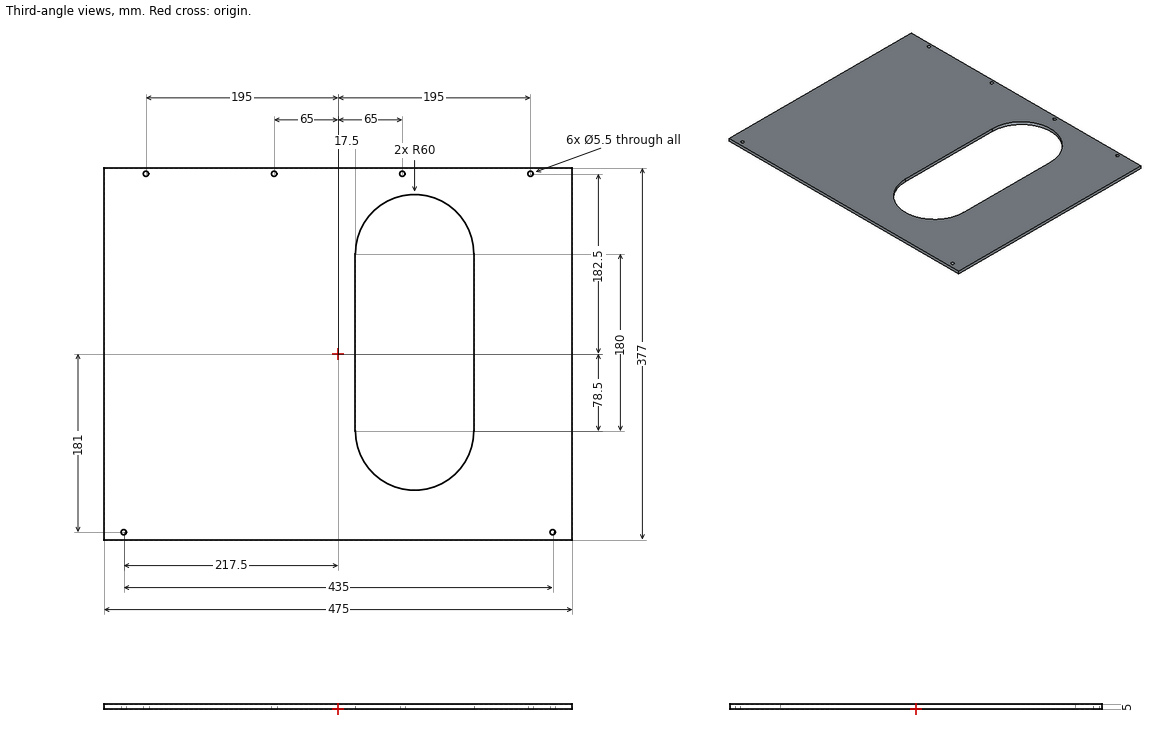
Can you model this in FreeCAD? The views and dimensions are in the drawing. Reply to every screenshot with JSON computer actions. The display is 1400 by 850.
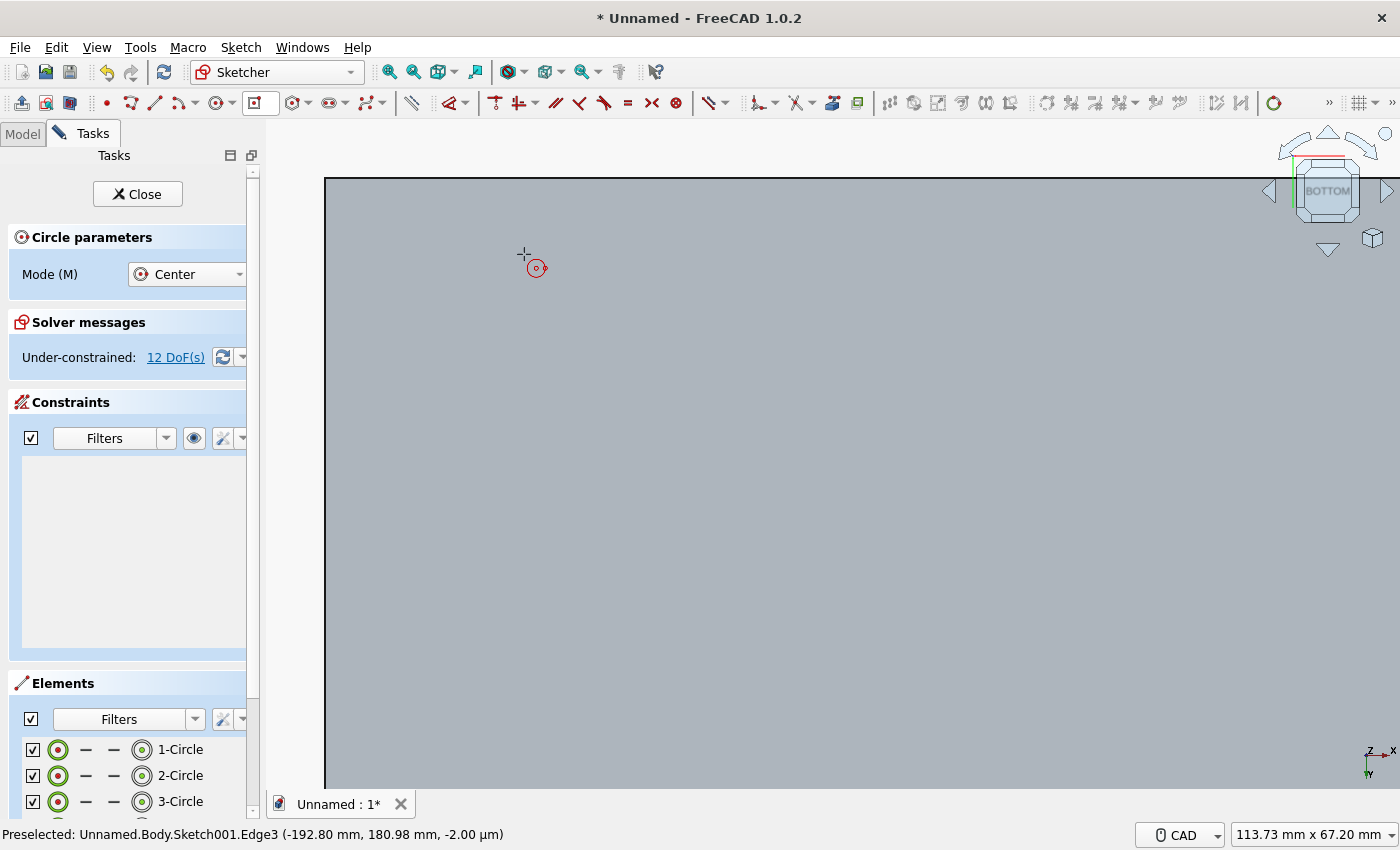
{"action": "scroll", "coordinate": [524, 253], "scroll_direction": "down", "scroll_amount": 11}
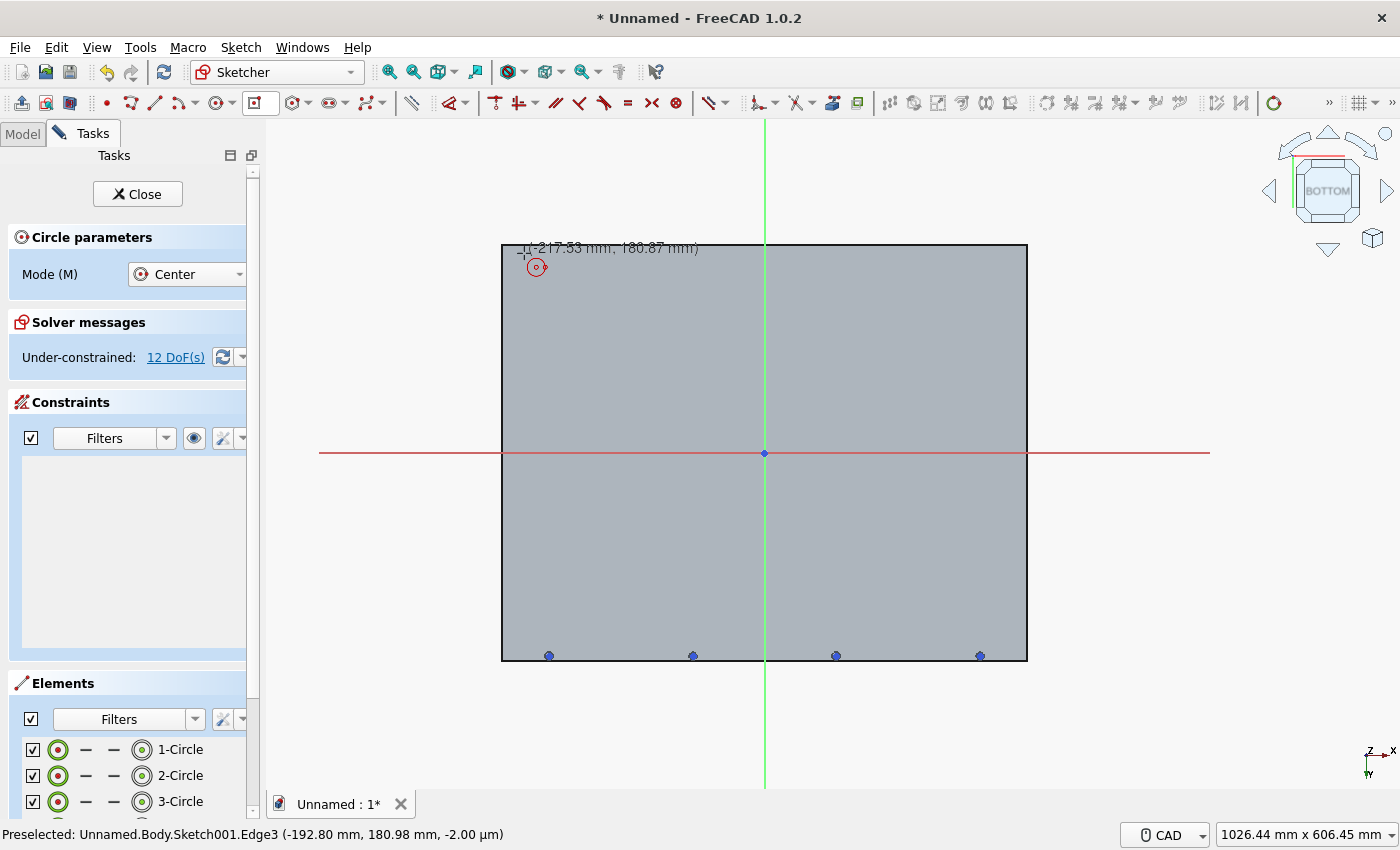
{"action": "left_click", "coordinate": [524, 253]}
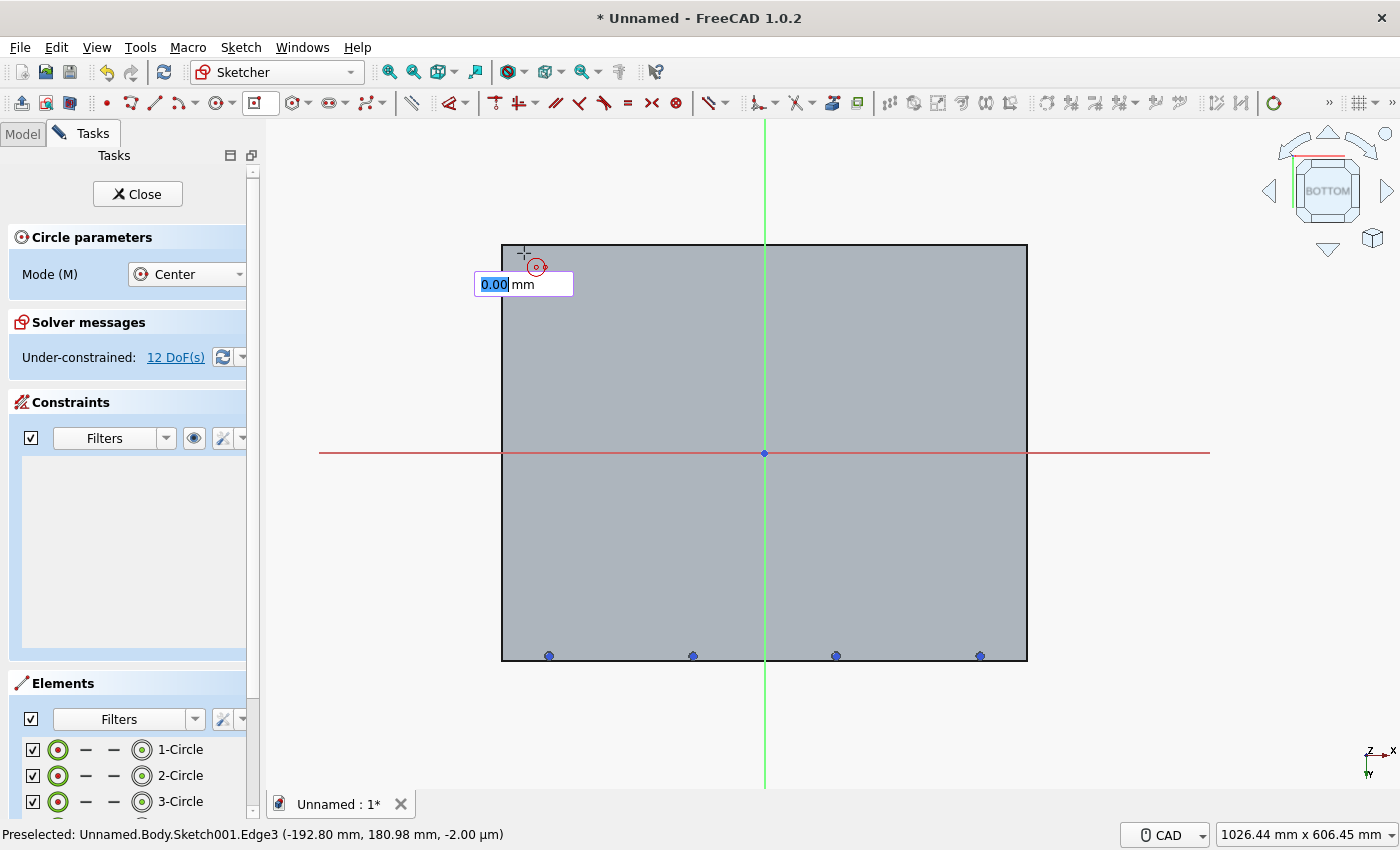
{"action": "scroll", "coordinate": [526, 251], "scroll_direction": "up", "scroll_amount": 9}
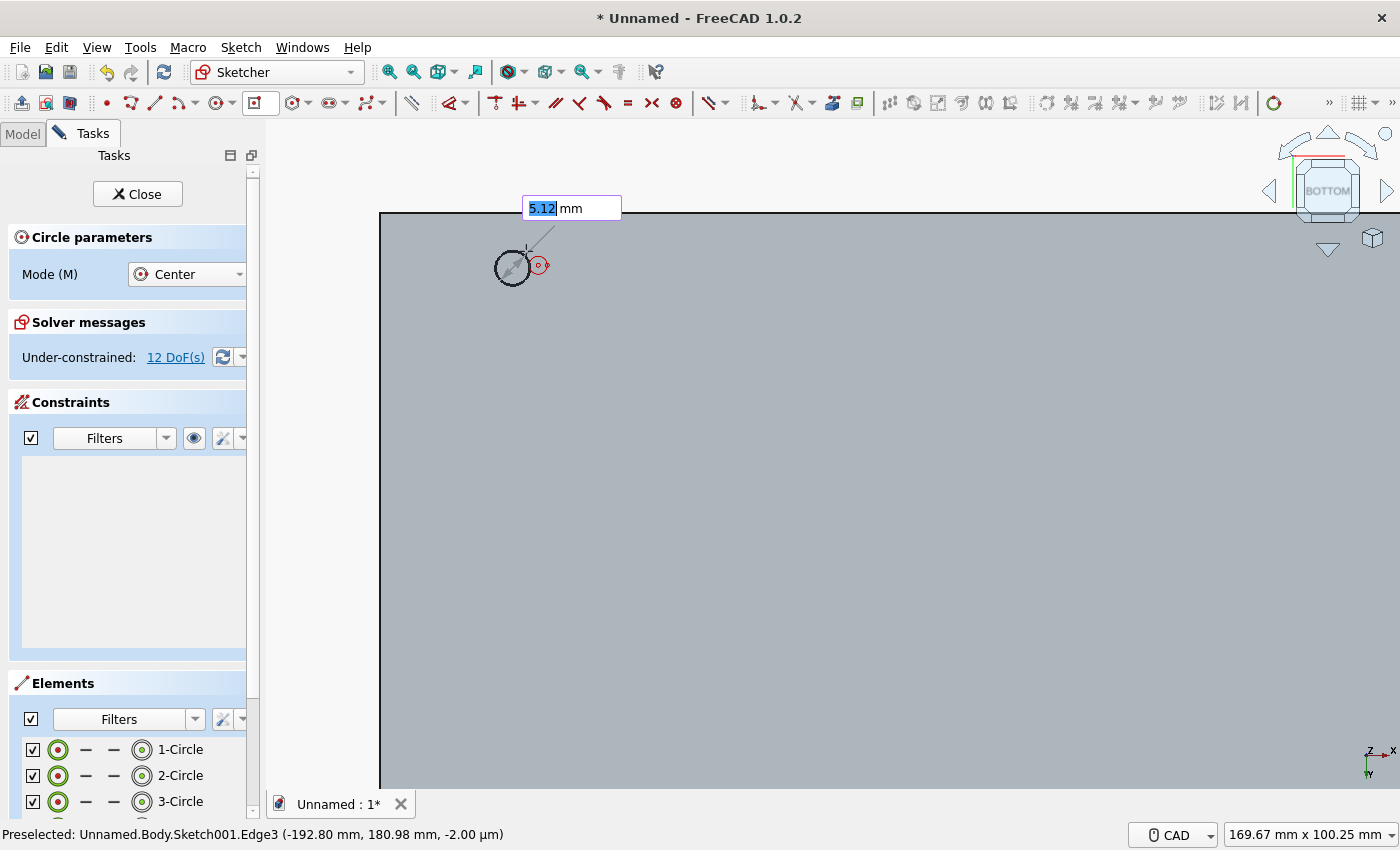
{"action": "left_click", "coordinate": [527, 250]}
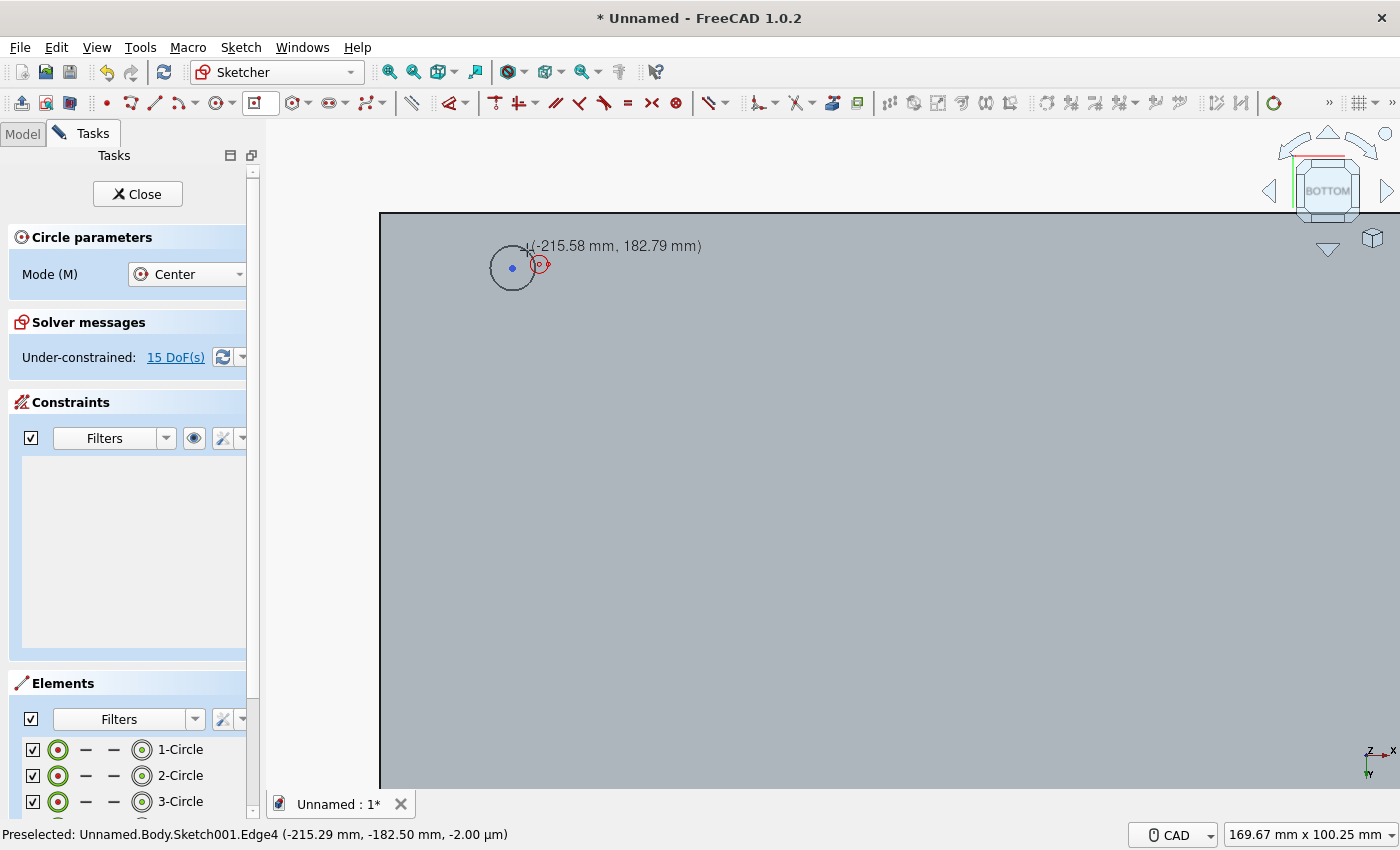
{"action": "scroll", "coordinate": [526, 251], "scroll_direction": "down", "scroll_amount": 9}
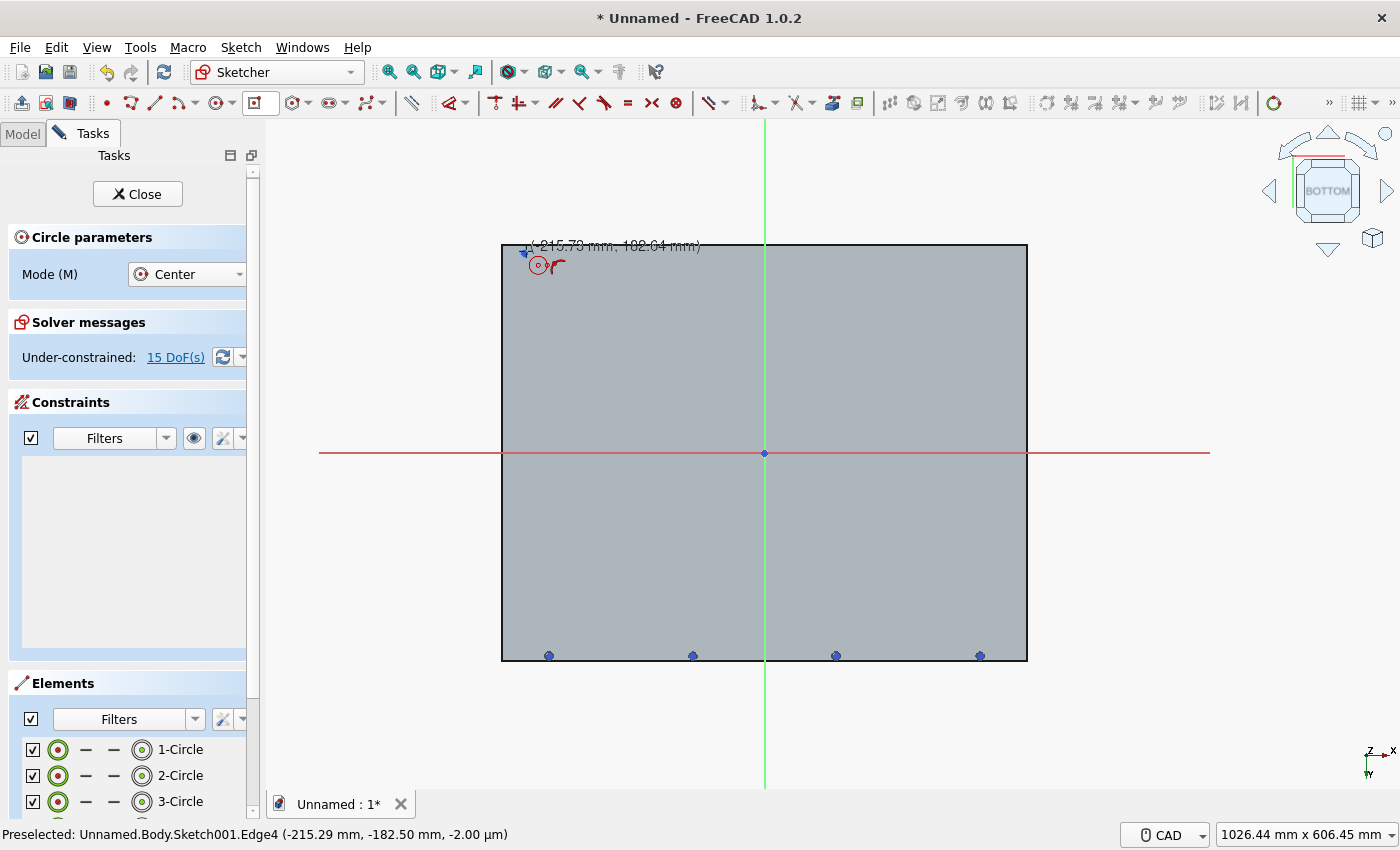
{"action": "scroll", "coordinate": [1005, 253], "scroll_direction": "up", "scroll_amount": 11}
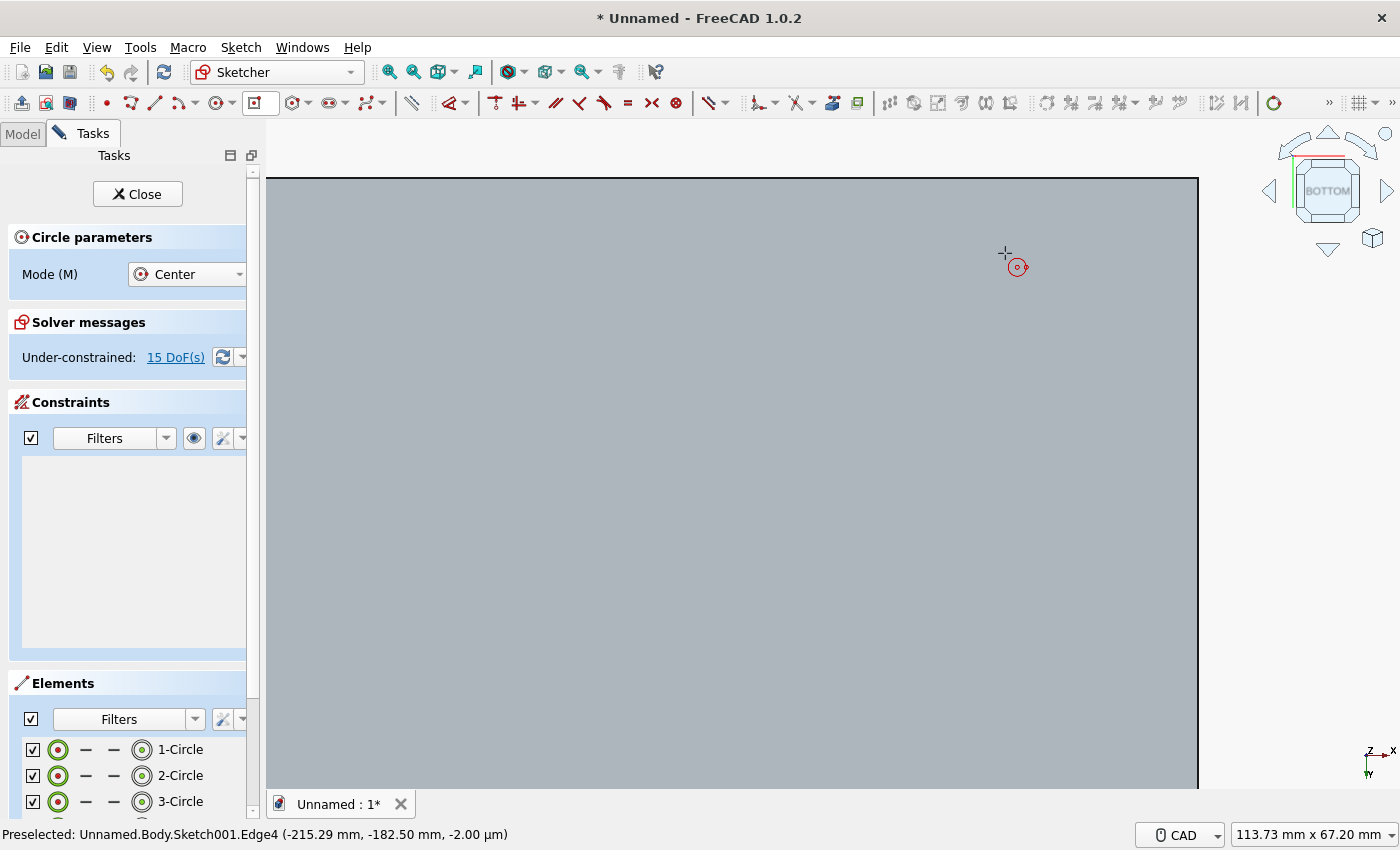
{"action": "scroll", "coordinate": [1006, 253], "scroll_direction": "down", "scroll_amount": 11}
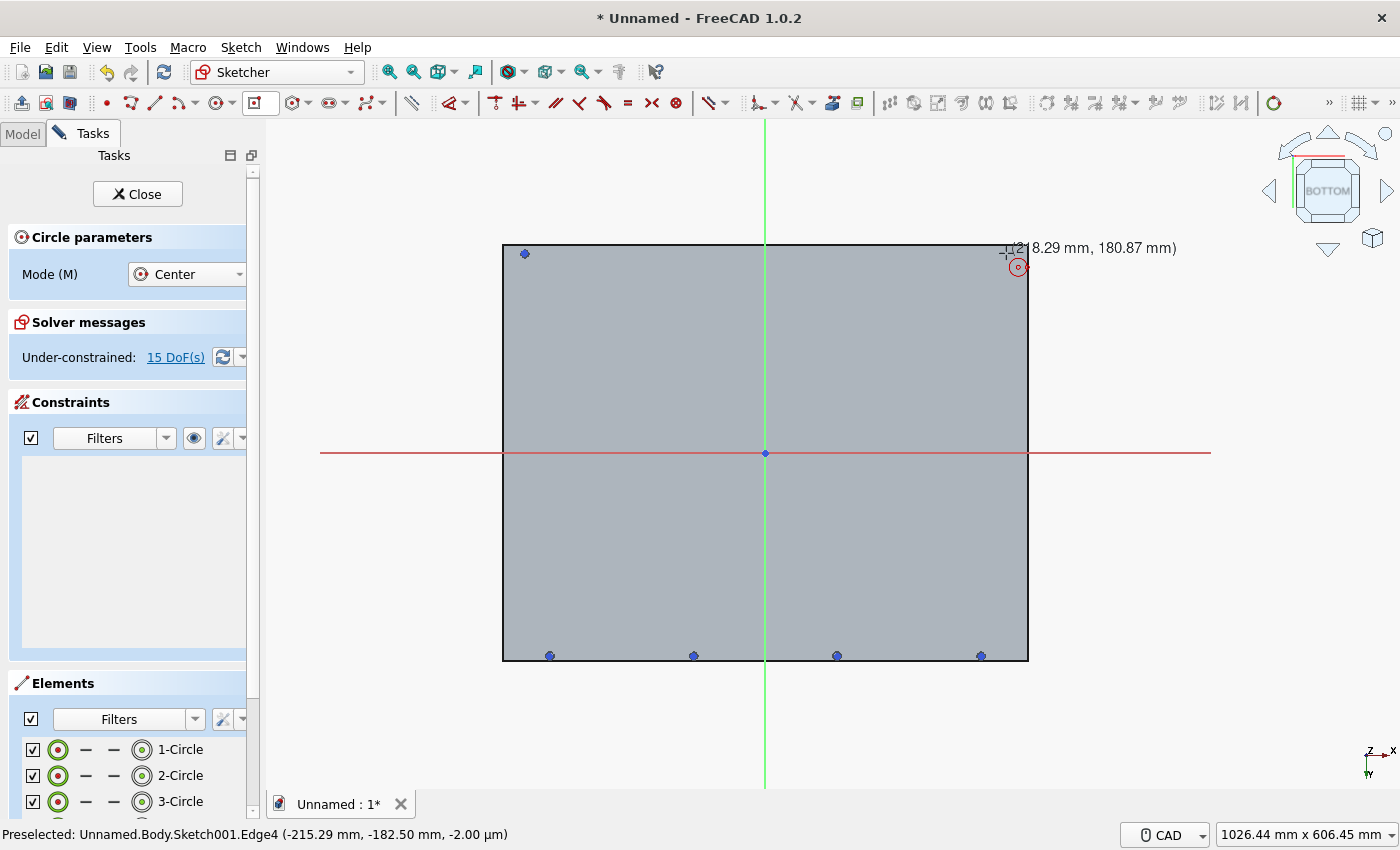
{"action": "left_click", "coordinate": [1006, 253]}